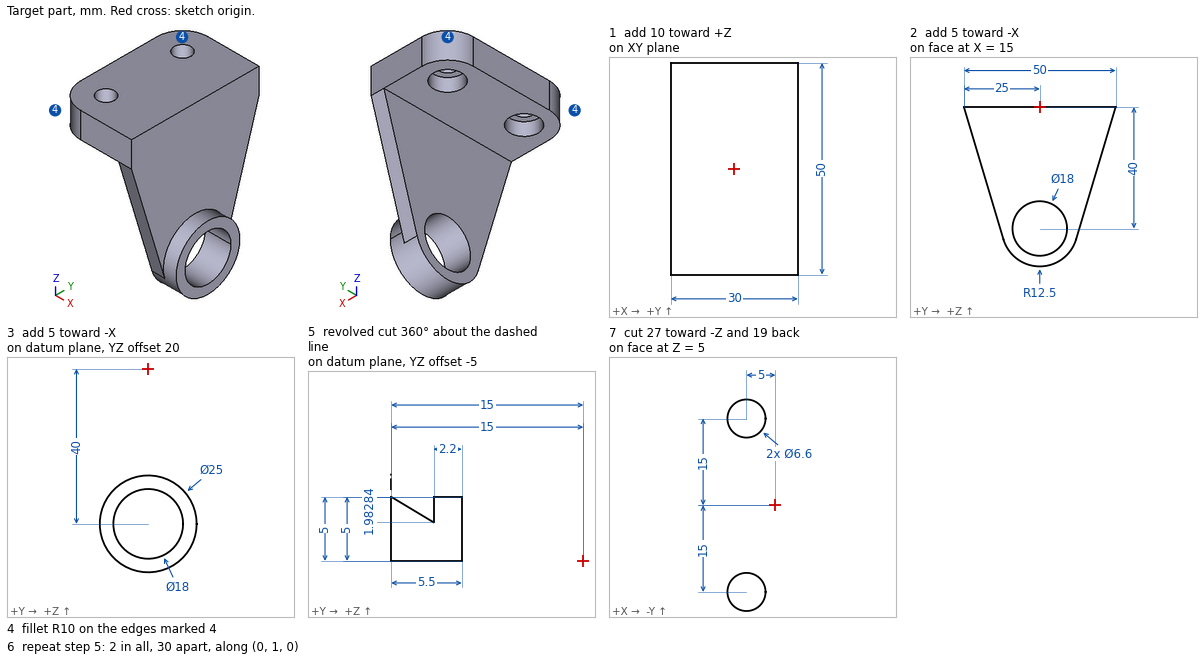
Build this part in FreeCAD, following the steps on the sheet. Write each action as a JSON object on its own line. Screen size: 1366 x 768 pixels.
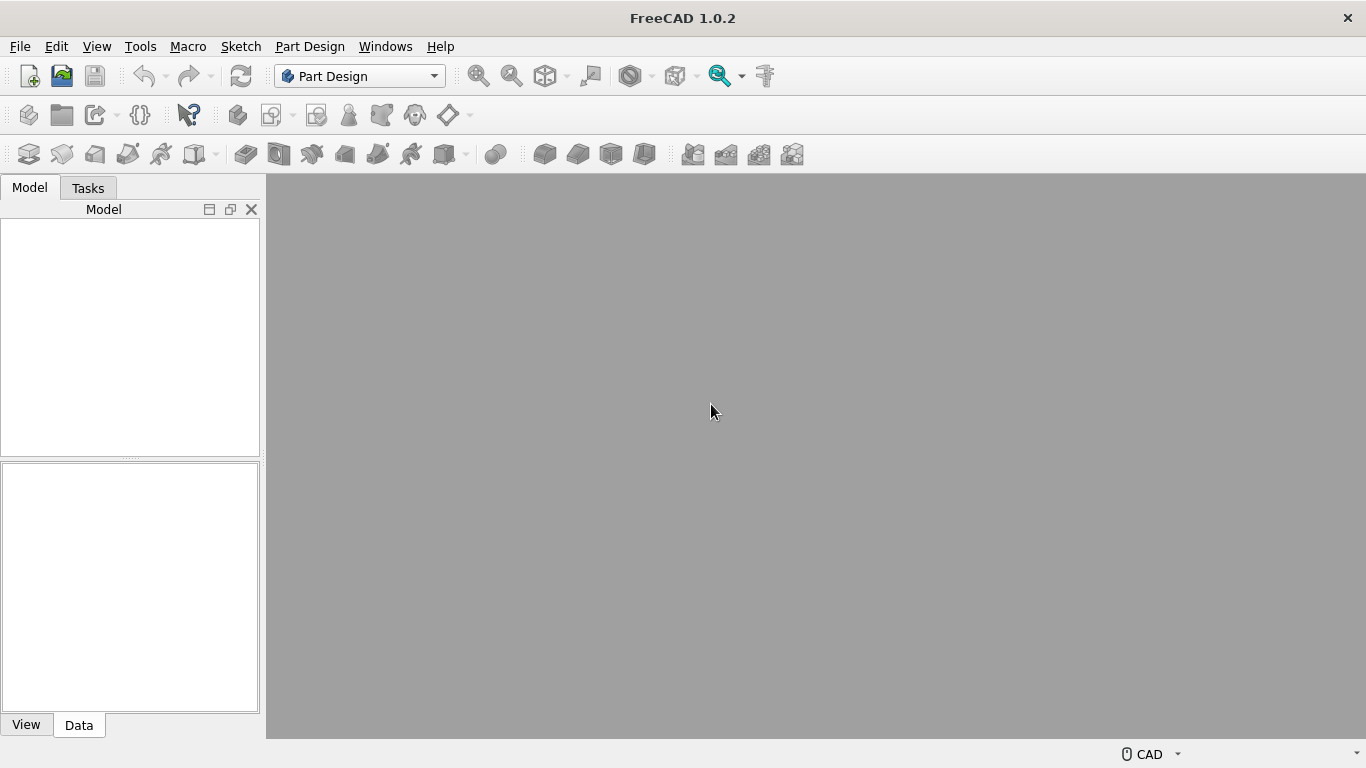
{"action": "left_click", "coordinate": [29, 76]}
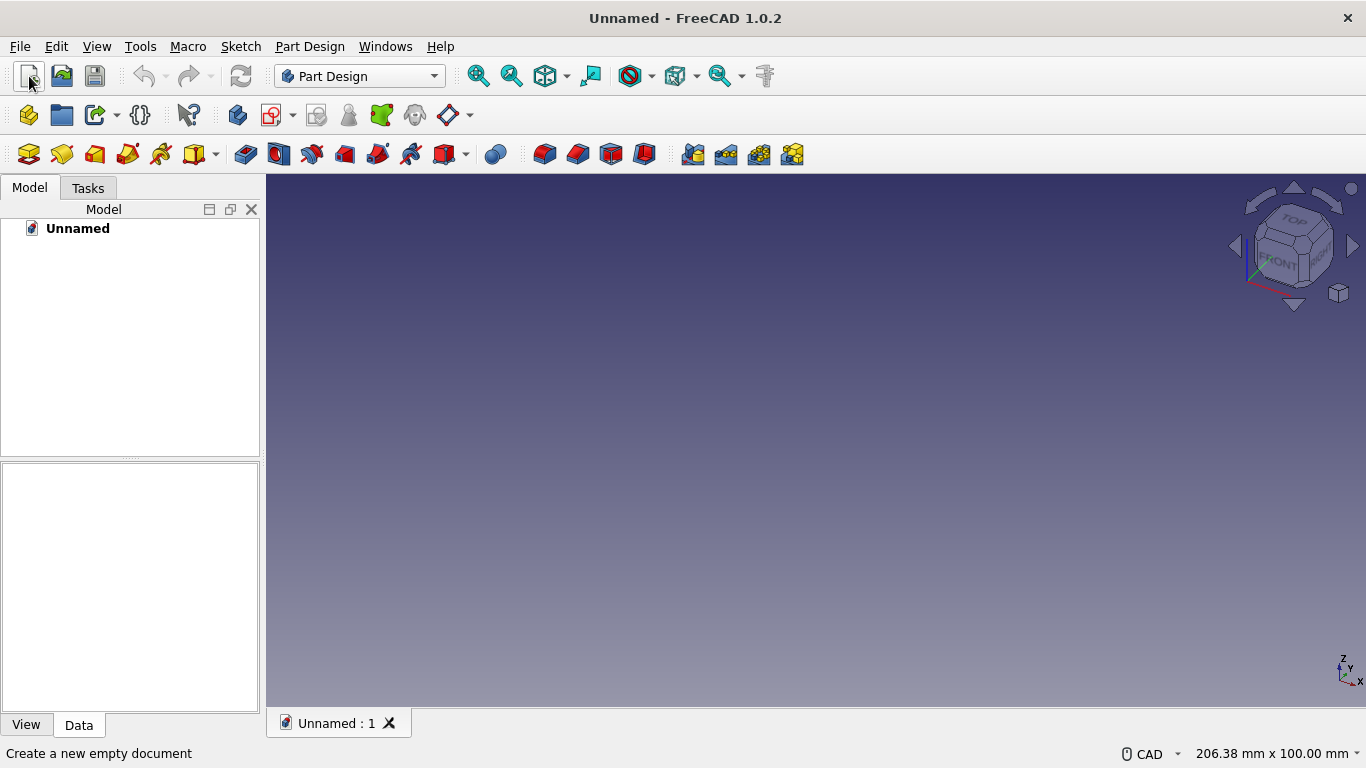
{"action": "left_click", "coordinate": [270, 116]}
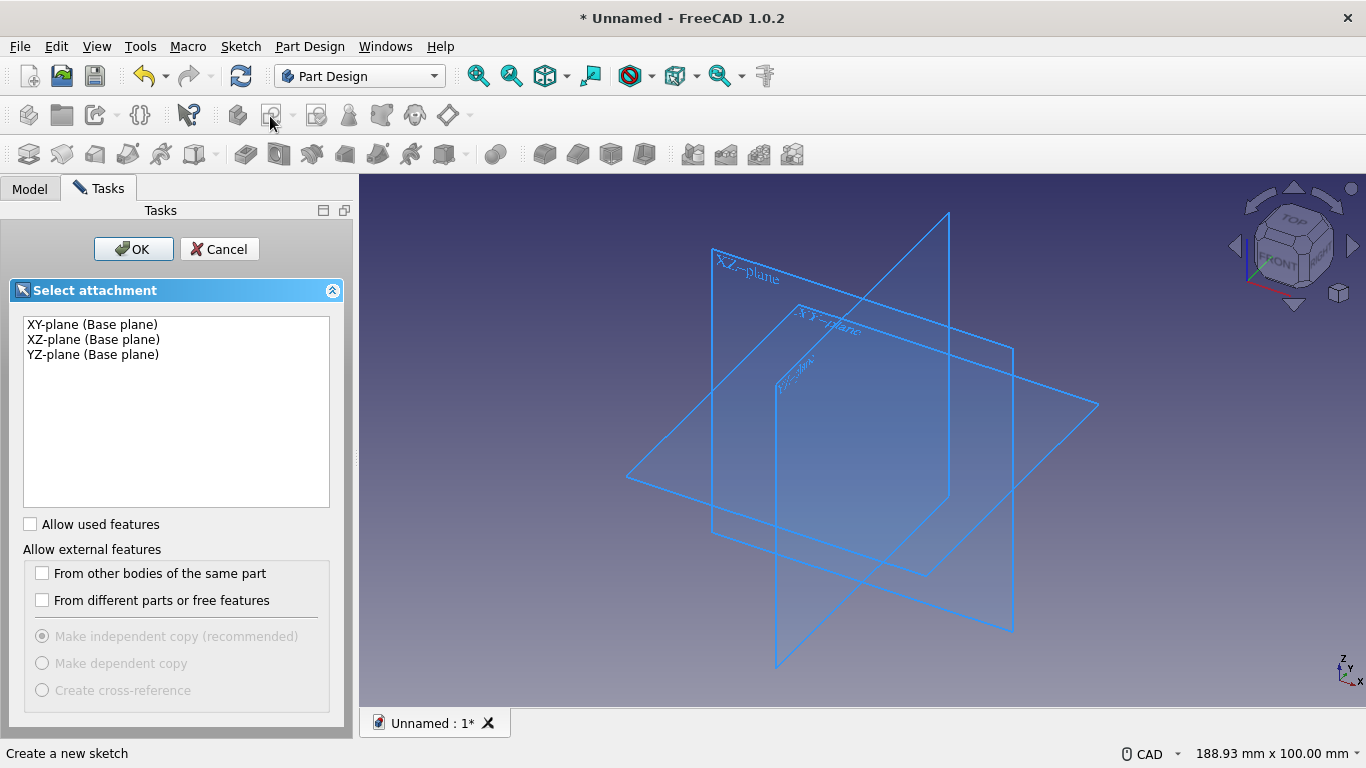
{"action": "left_click", "coordinate": [84, 324]}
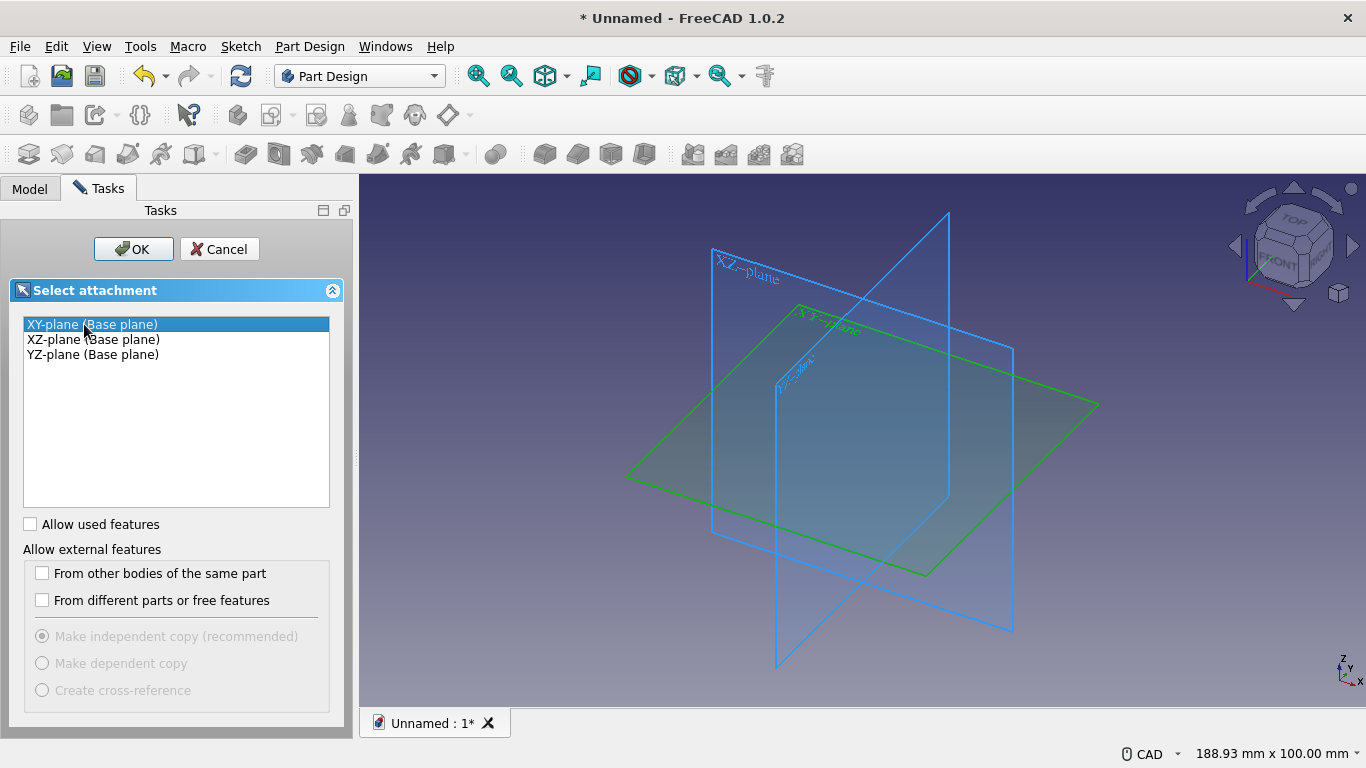
{"action": "left_click", "coordinate": [134, 249]}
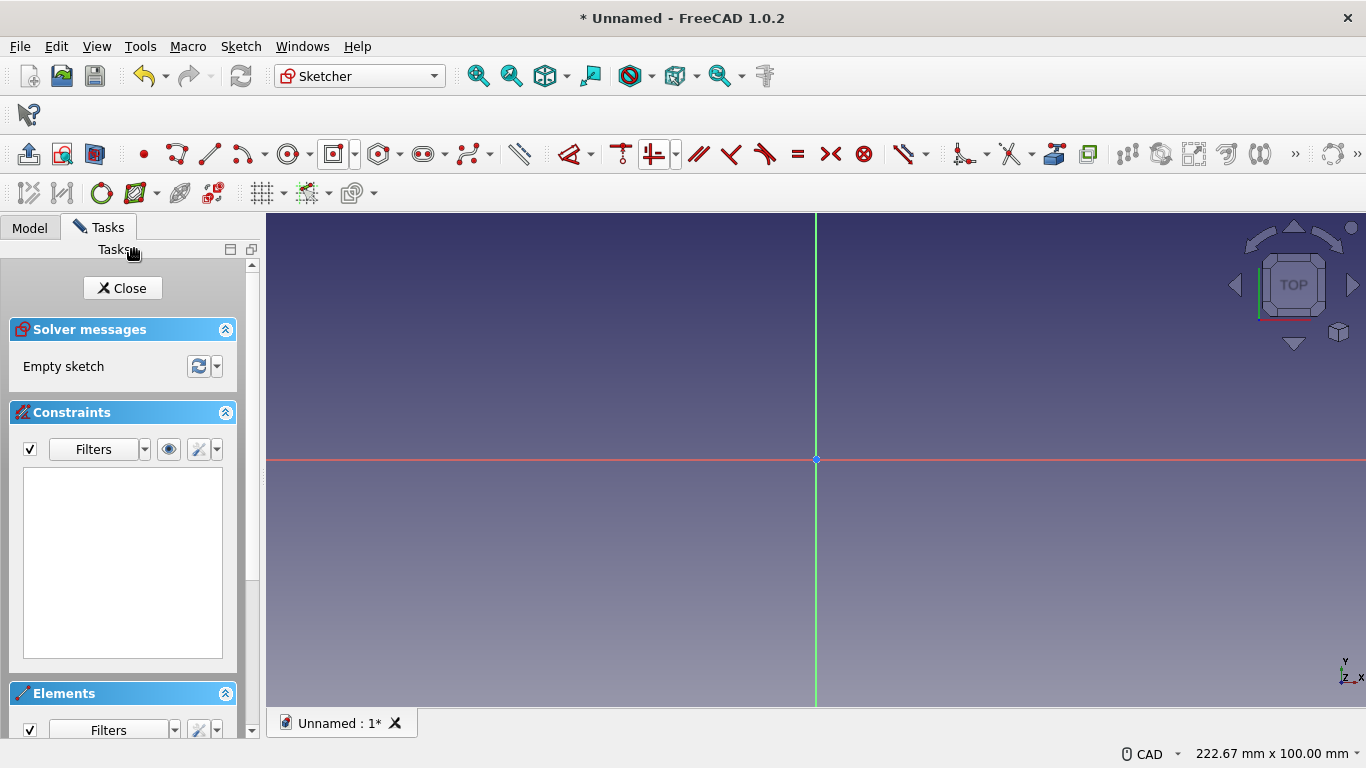
{"action": "key", "text": "g v"}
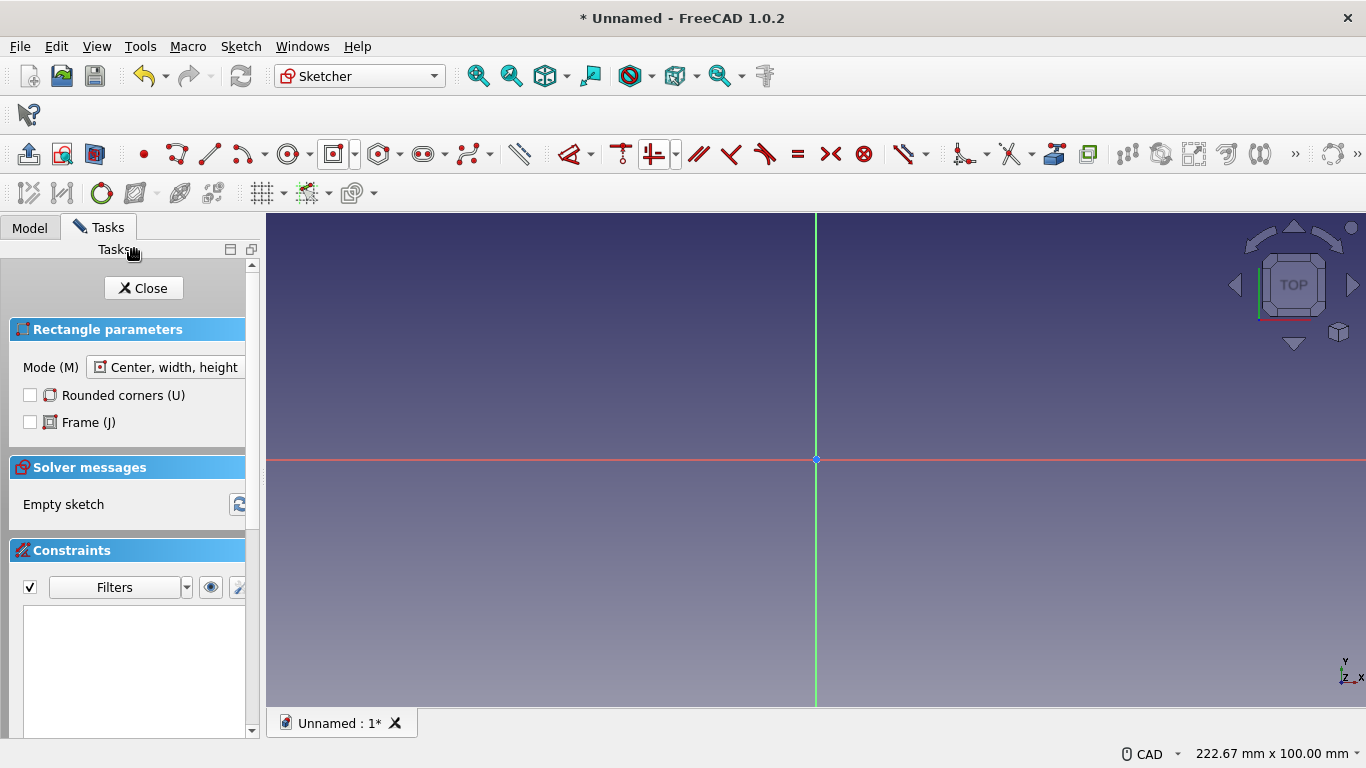
{"action": "left_click", "coordinate": [816, 460]}
{"action": "mouse_move", "coordinate": [890, 336]}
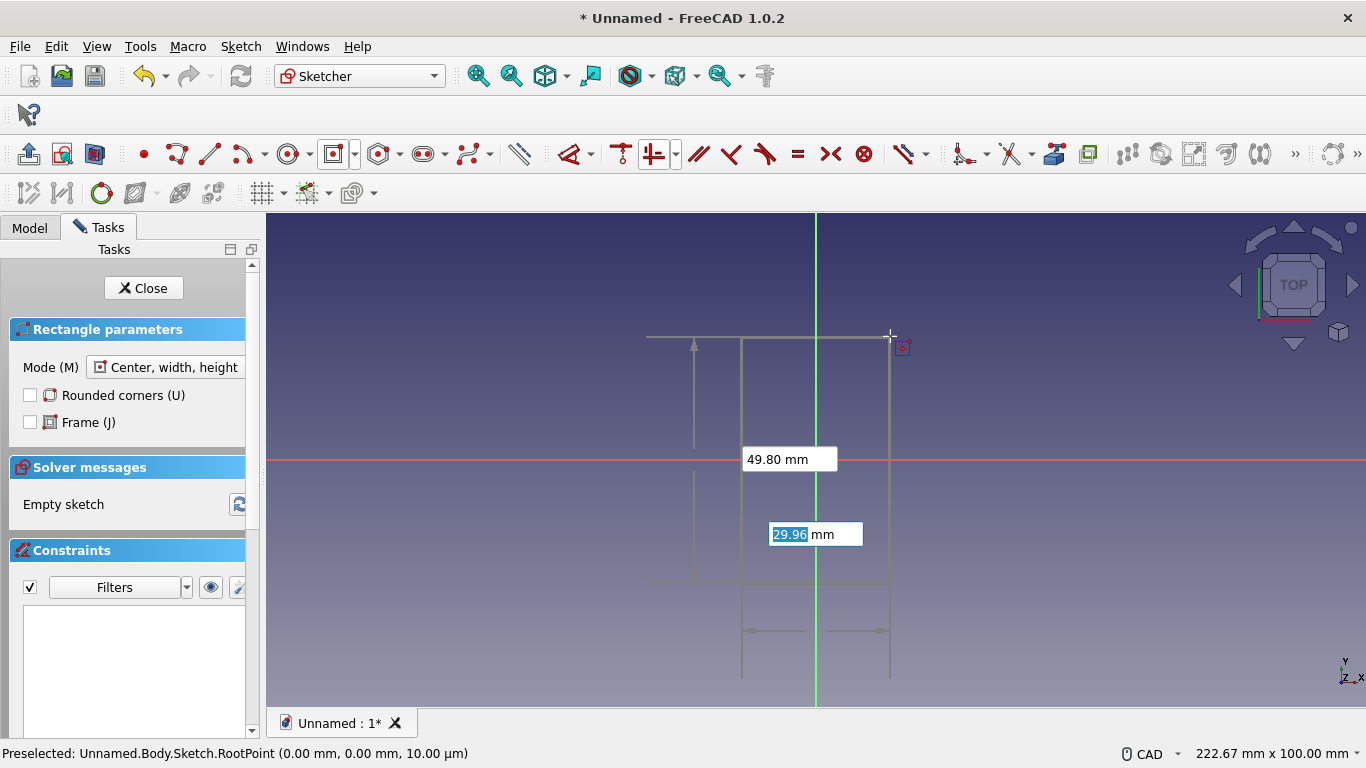
{"action": "type", "text": "30"}
{"action": "key", "text": "Tab"}
{"action": "type", "text": "50"}
{"action": "key", "text": "Return"}
{"action": "key", "text": "Escape"}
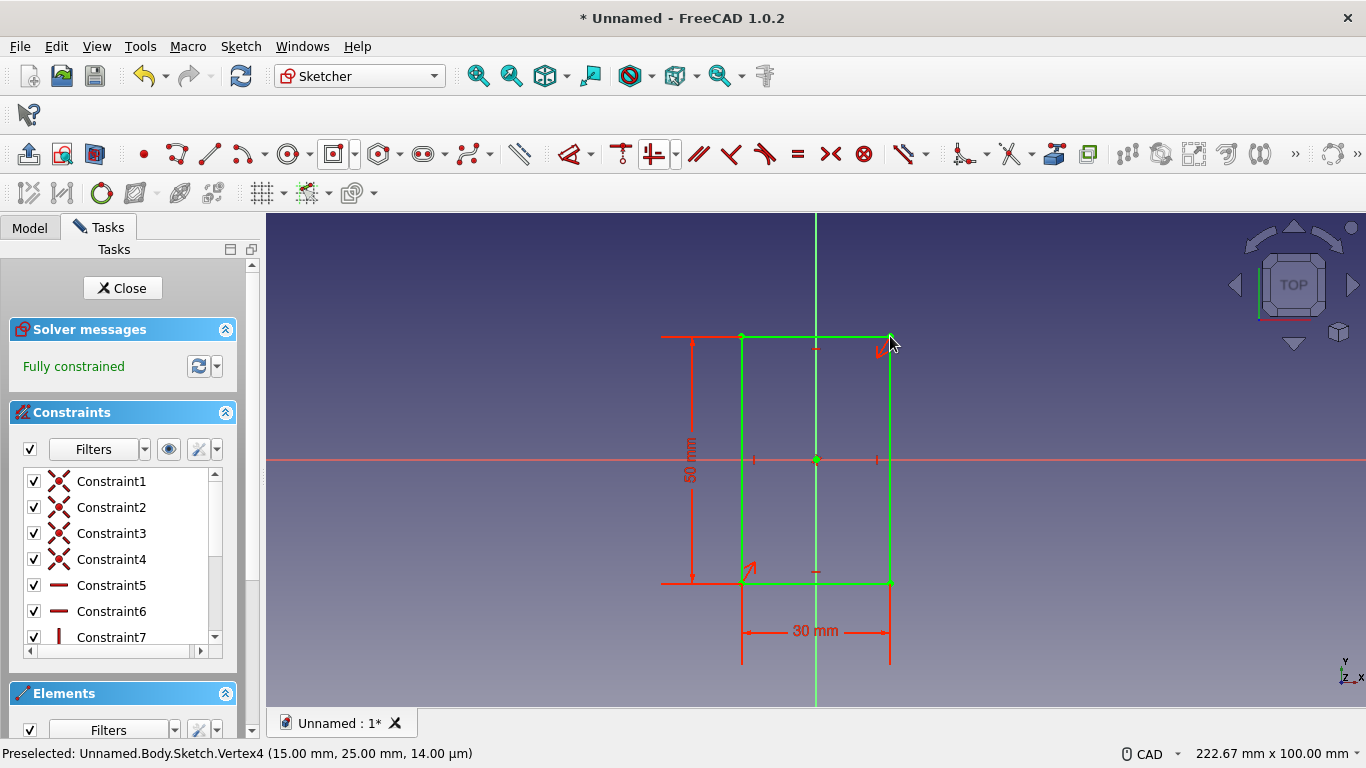
{"action": "left_click", "coordinate": [123, 288]}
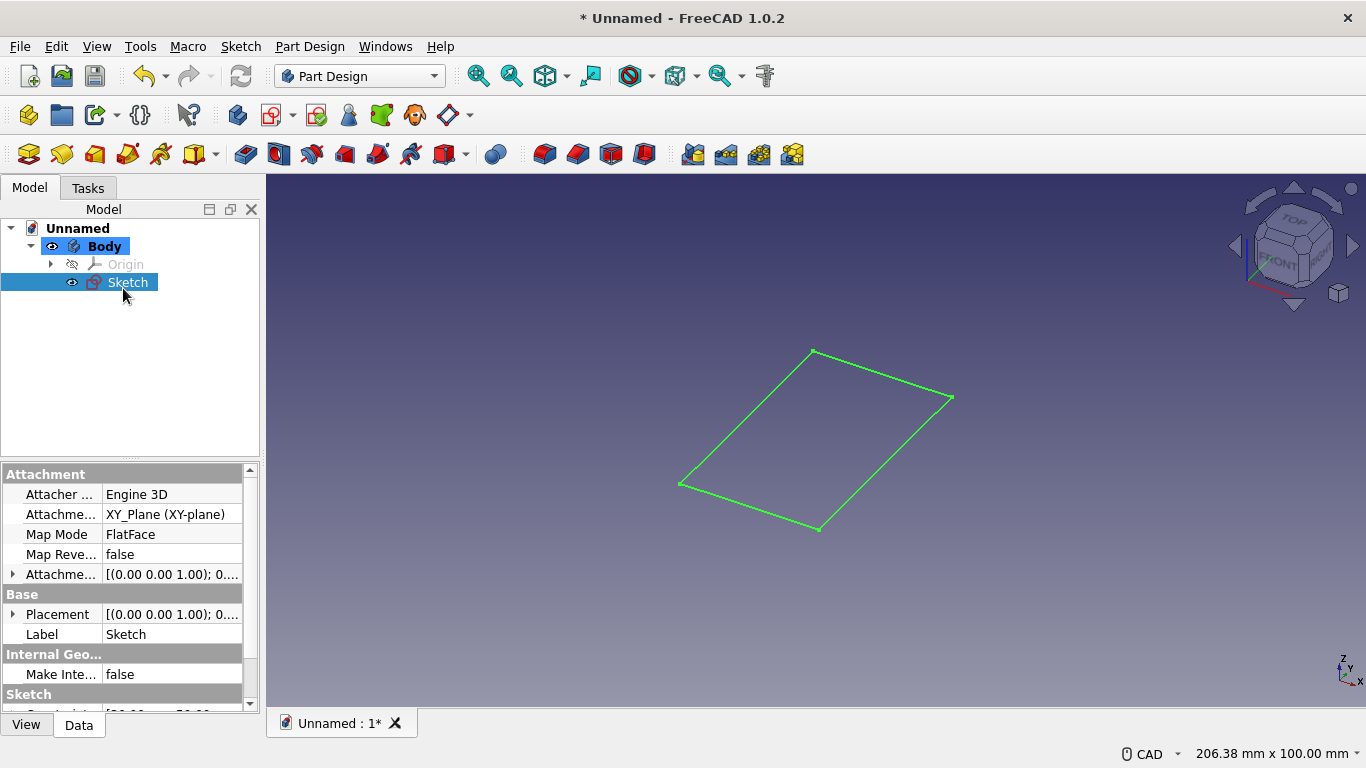
{"action": "left_click", "coordinate": [29, 154]}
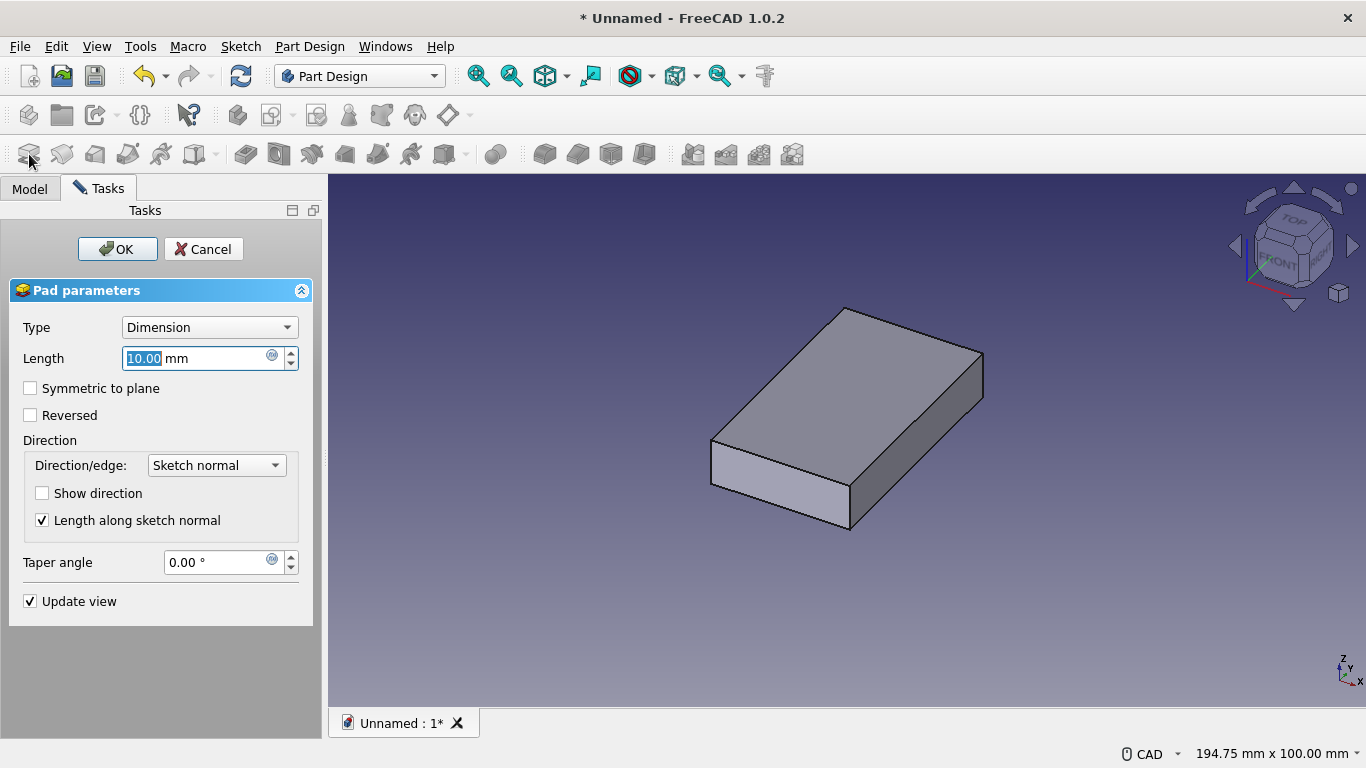
{"action": "type", "text": "10"}
{"action": "key", "text": "Tab"}